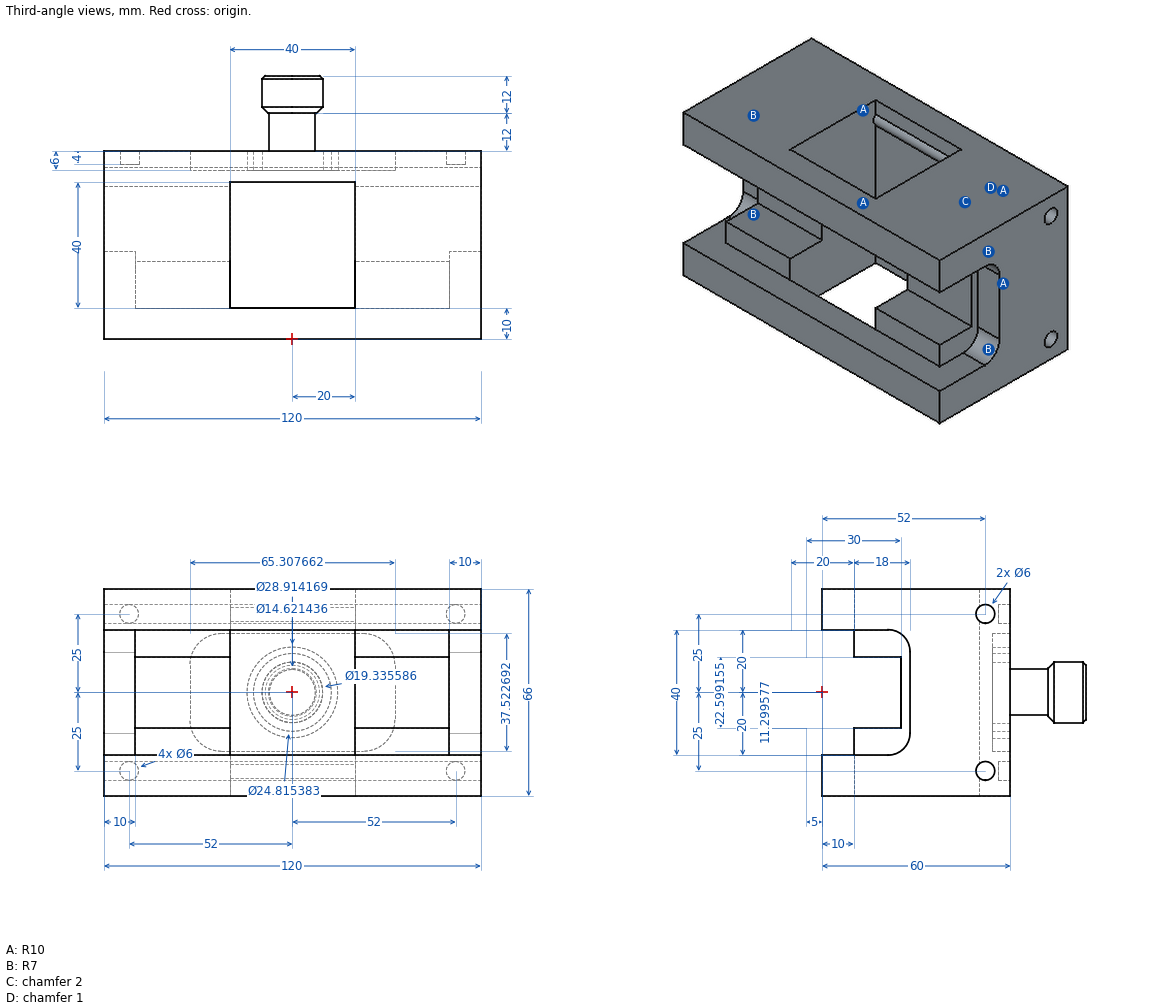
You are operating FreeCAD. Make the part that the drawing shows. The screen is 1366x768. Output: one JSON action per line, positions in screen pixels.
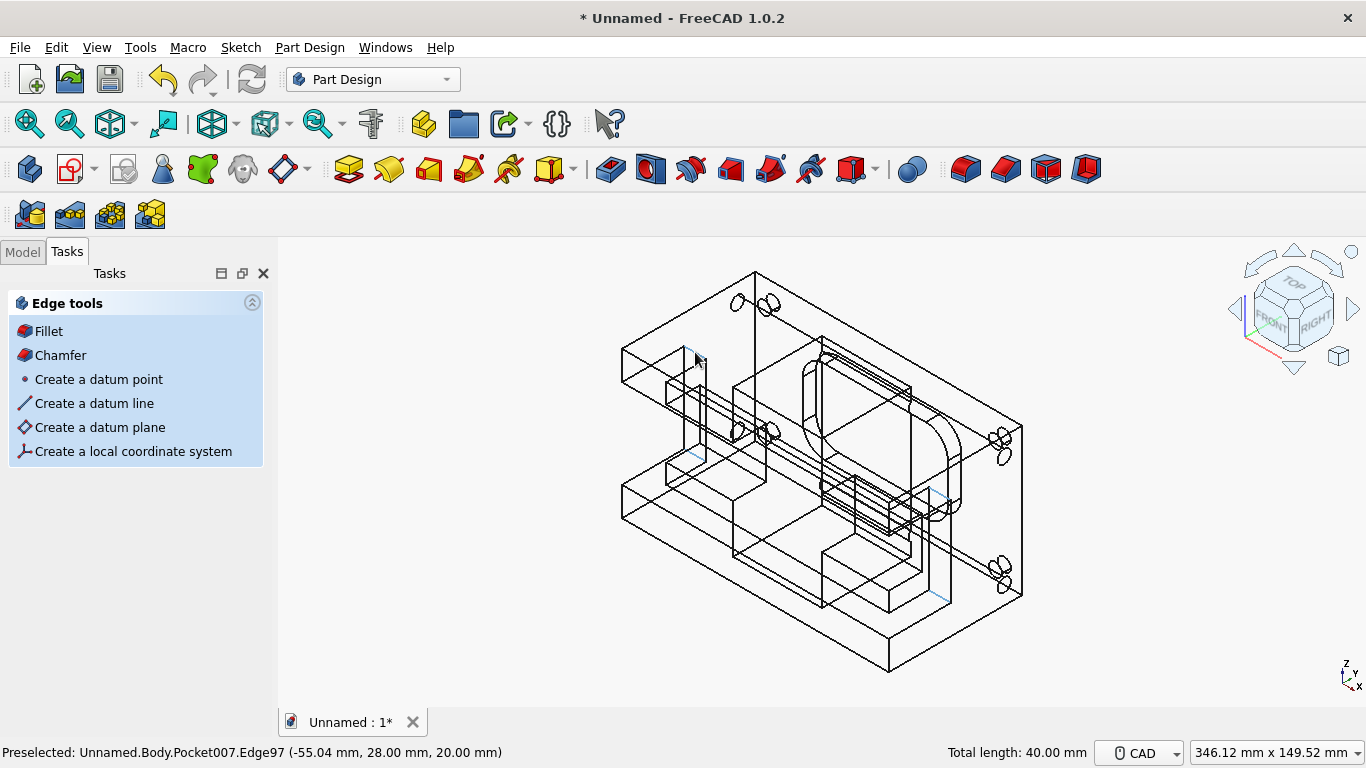
{"action": "key", "text": "v 1"}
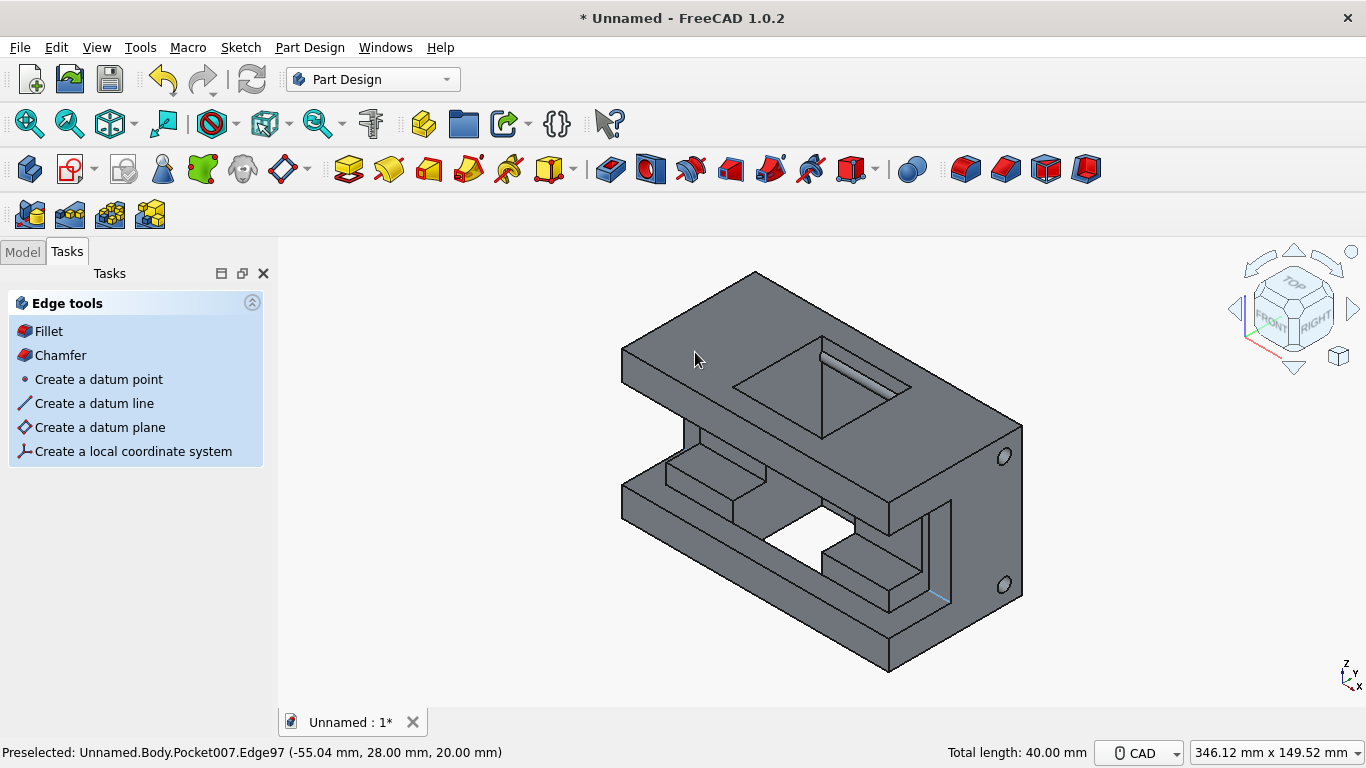
{"action": "left_click", "coordinate": [966, 170]}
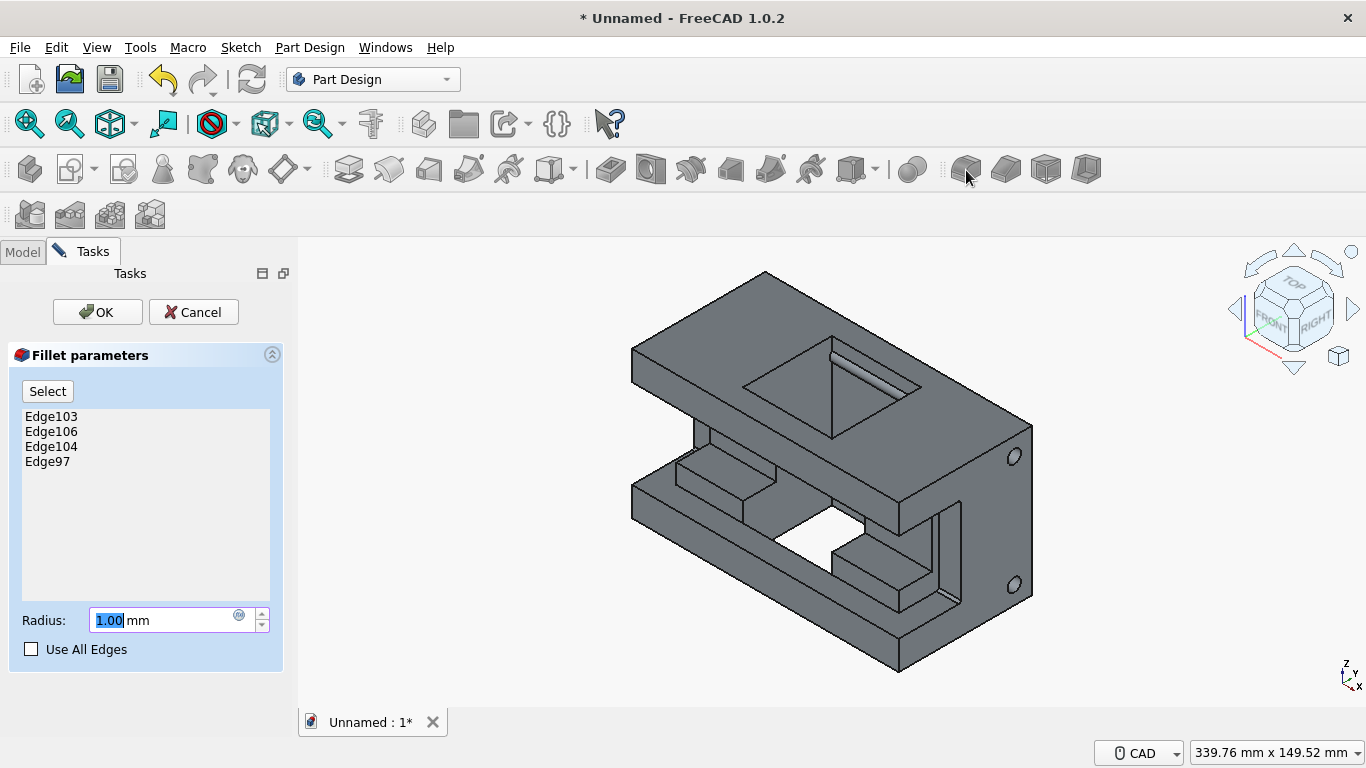
{"action": "type", "text": "7"}
{"action": "key", "text": "Tab"}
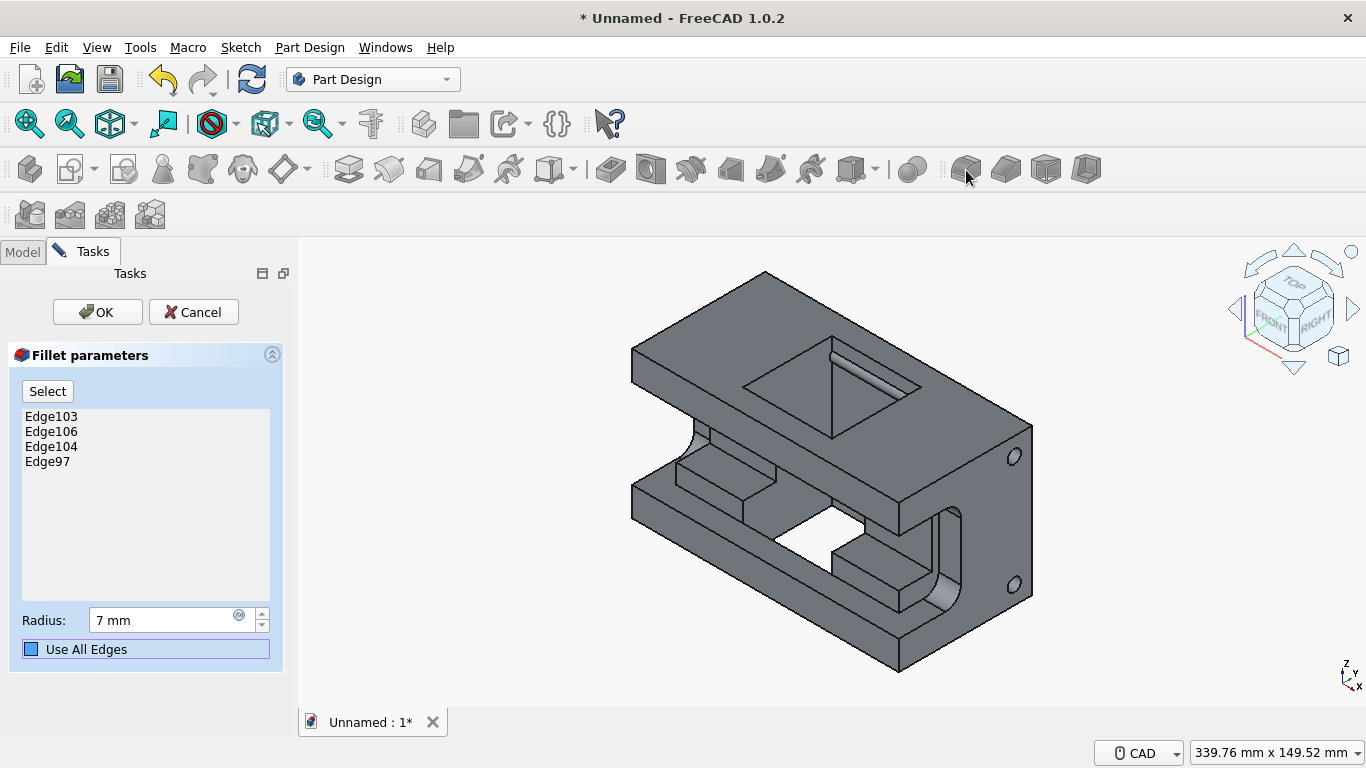
{"action": "left_click", "coordinate": [98, 312]}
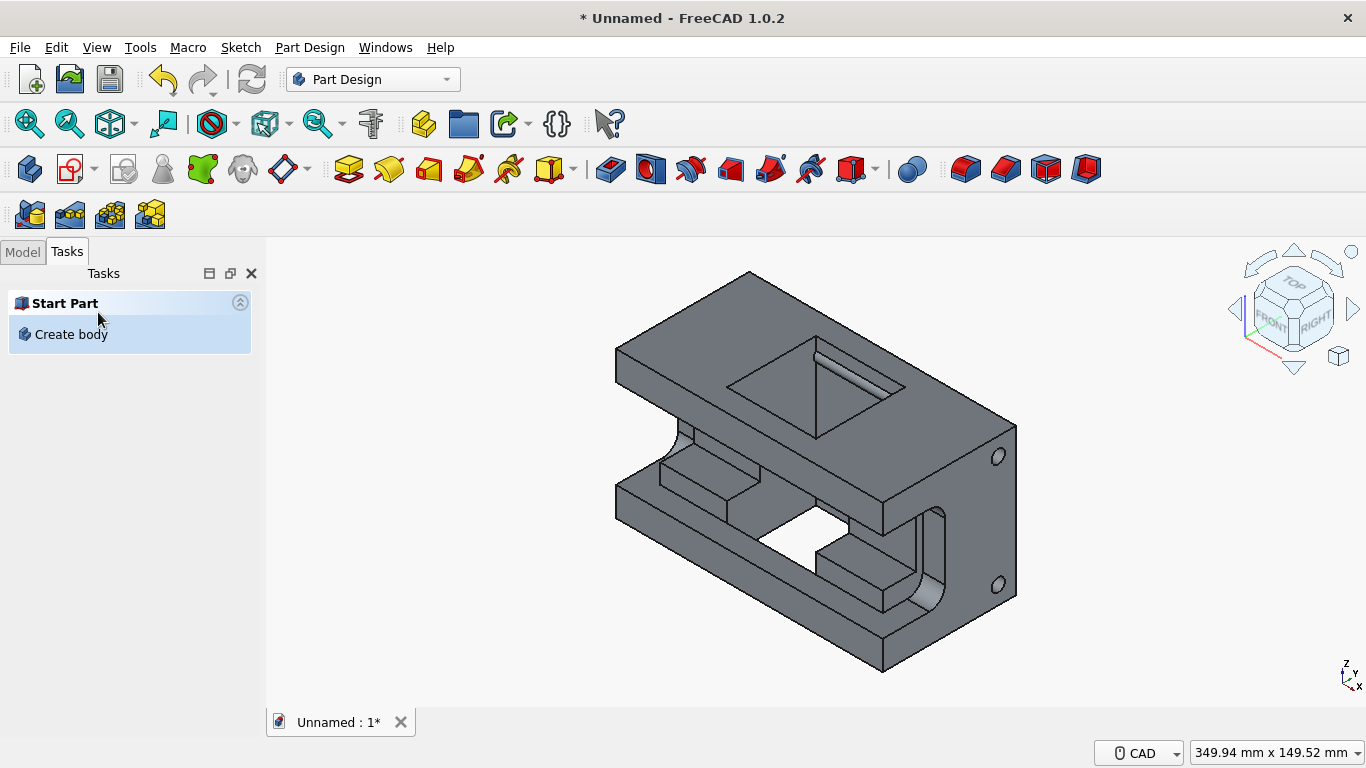
{"action": "key", "text": "4"}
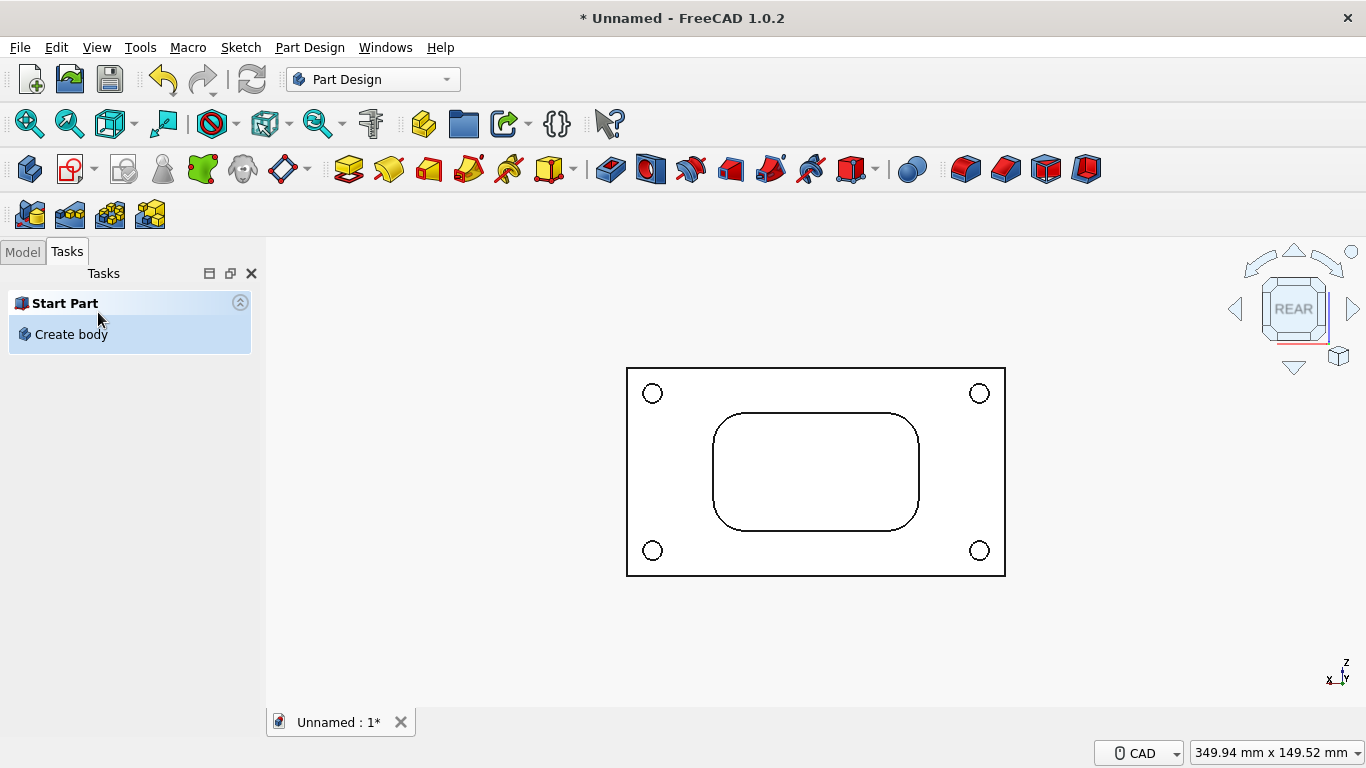
{"action": "left_click", "coordinate": [30, 124]}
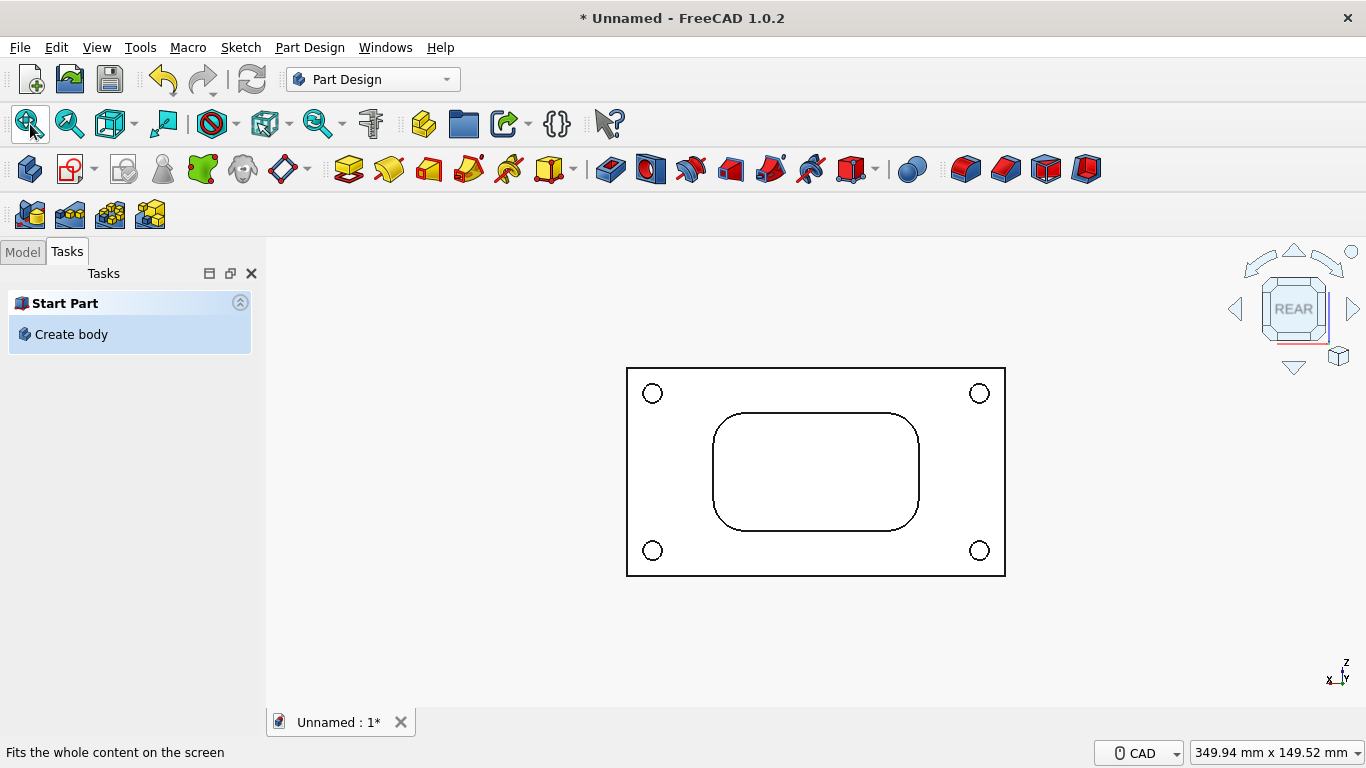
{"action": "left_click", "coordinate": [787, 471]}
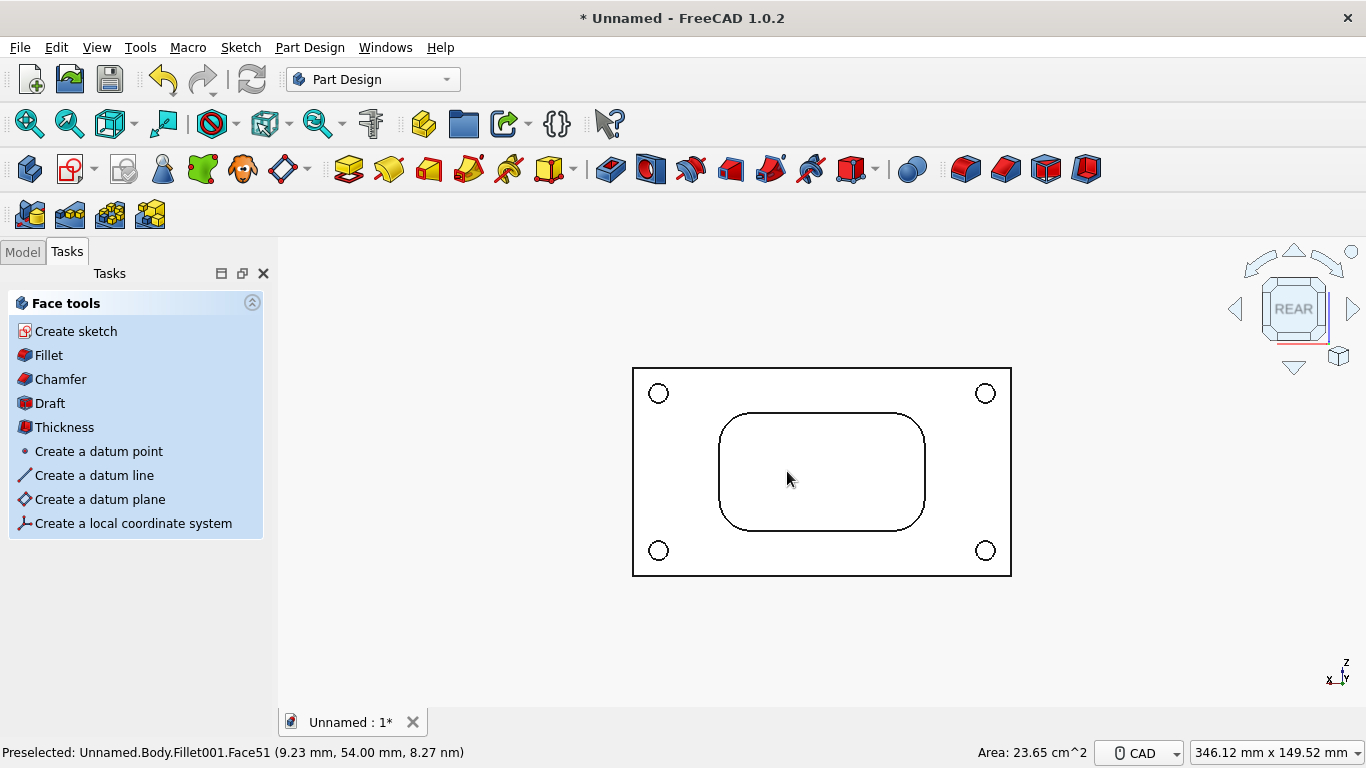
{"action": "left_click", "coordinate": [70, 170]}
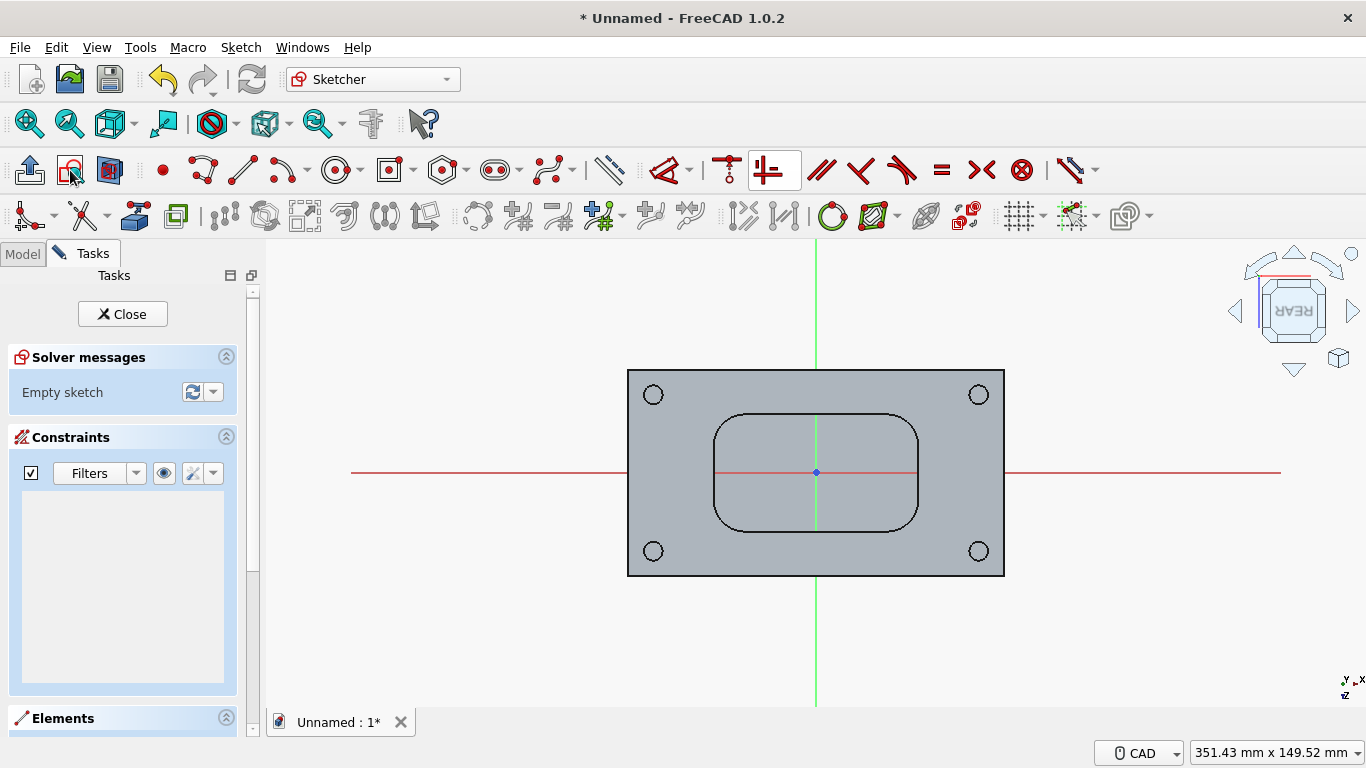
{"action": "left_click", "coordinate": [110, 170]}